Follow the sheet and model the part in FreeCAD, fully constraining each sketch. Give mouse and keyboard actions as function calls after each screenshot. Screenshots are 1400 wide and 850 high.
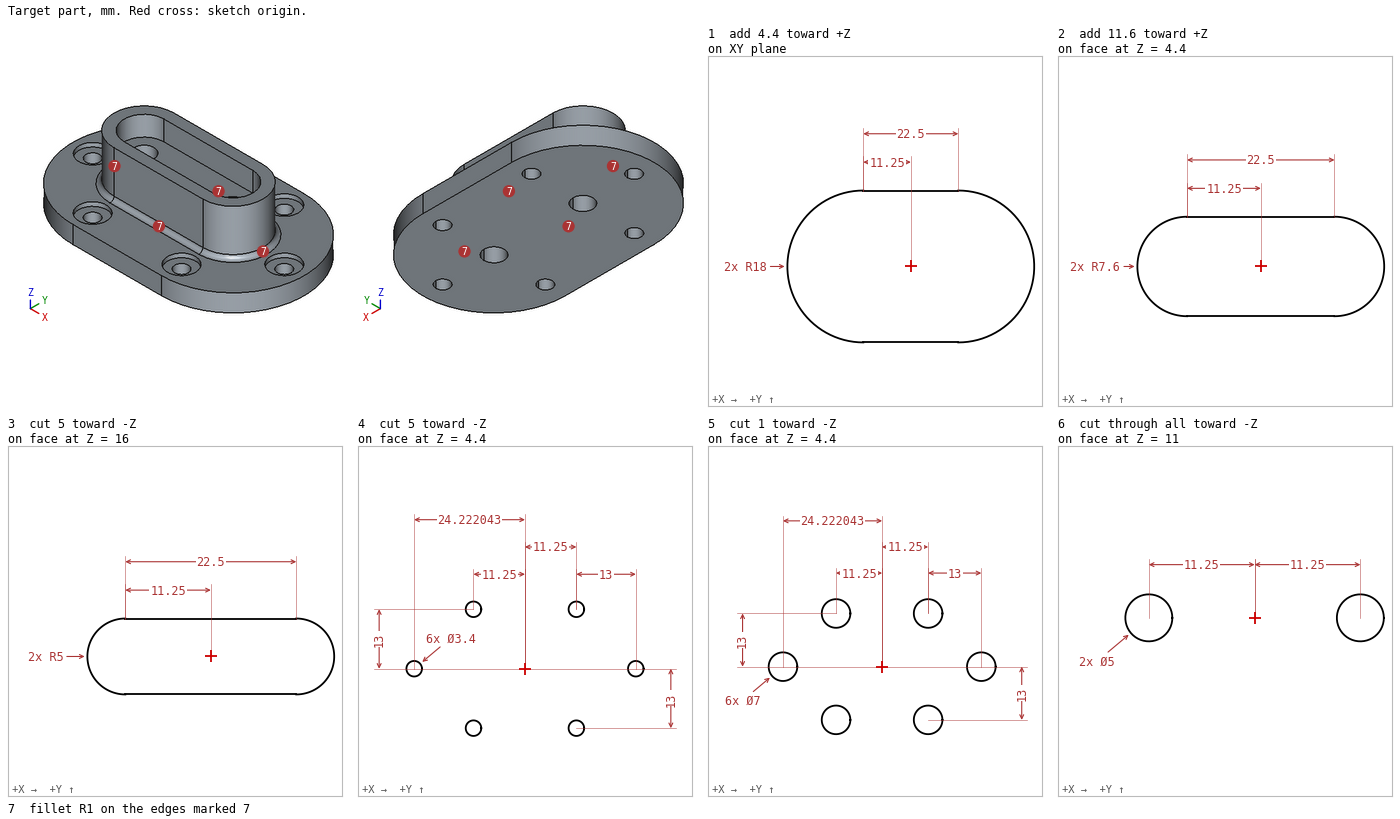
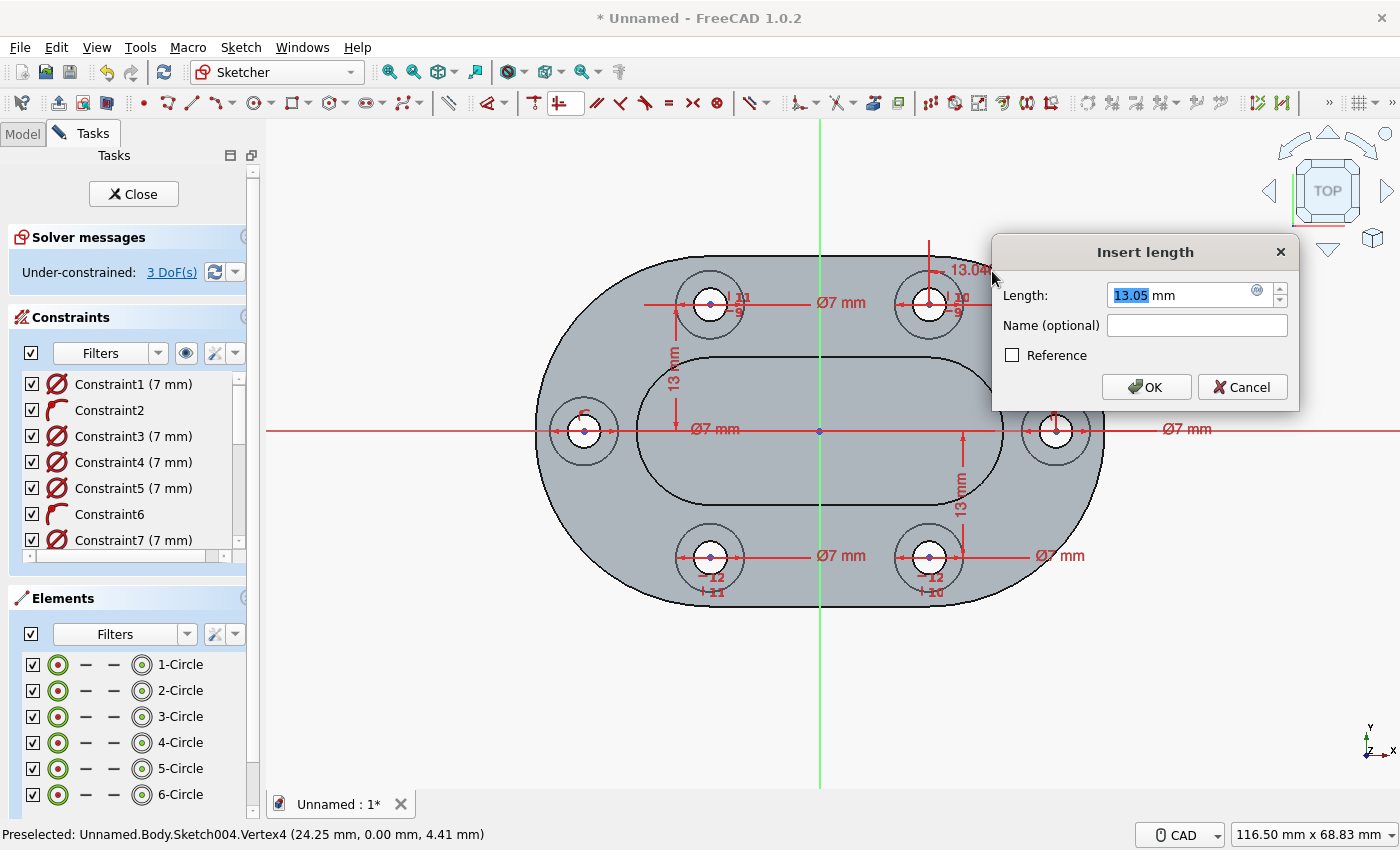
text(13)
key(Return)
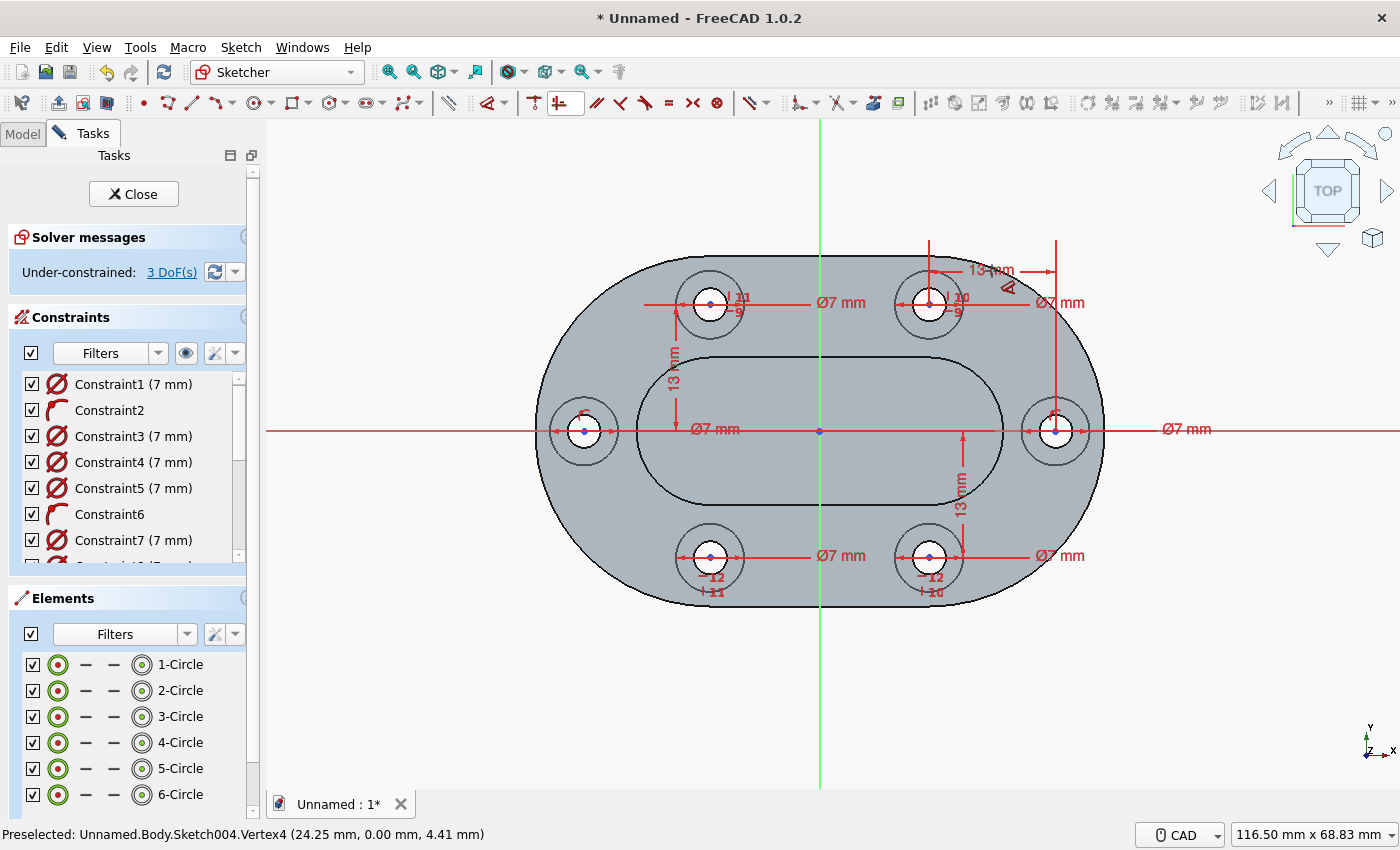
click(710, 305)
click(765, 271)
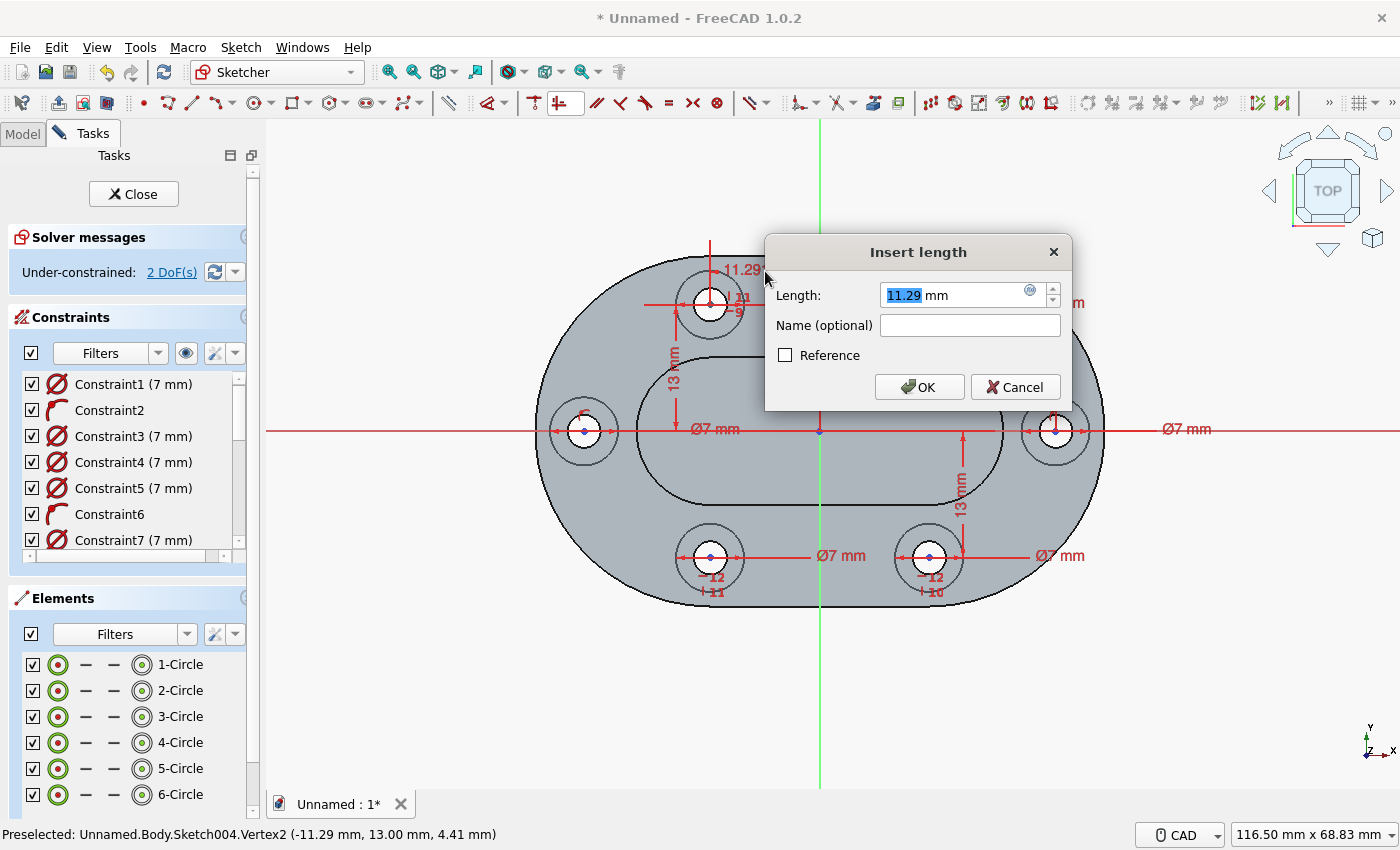
text(11.25)
key(Return)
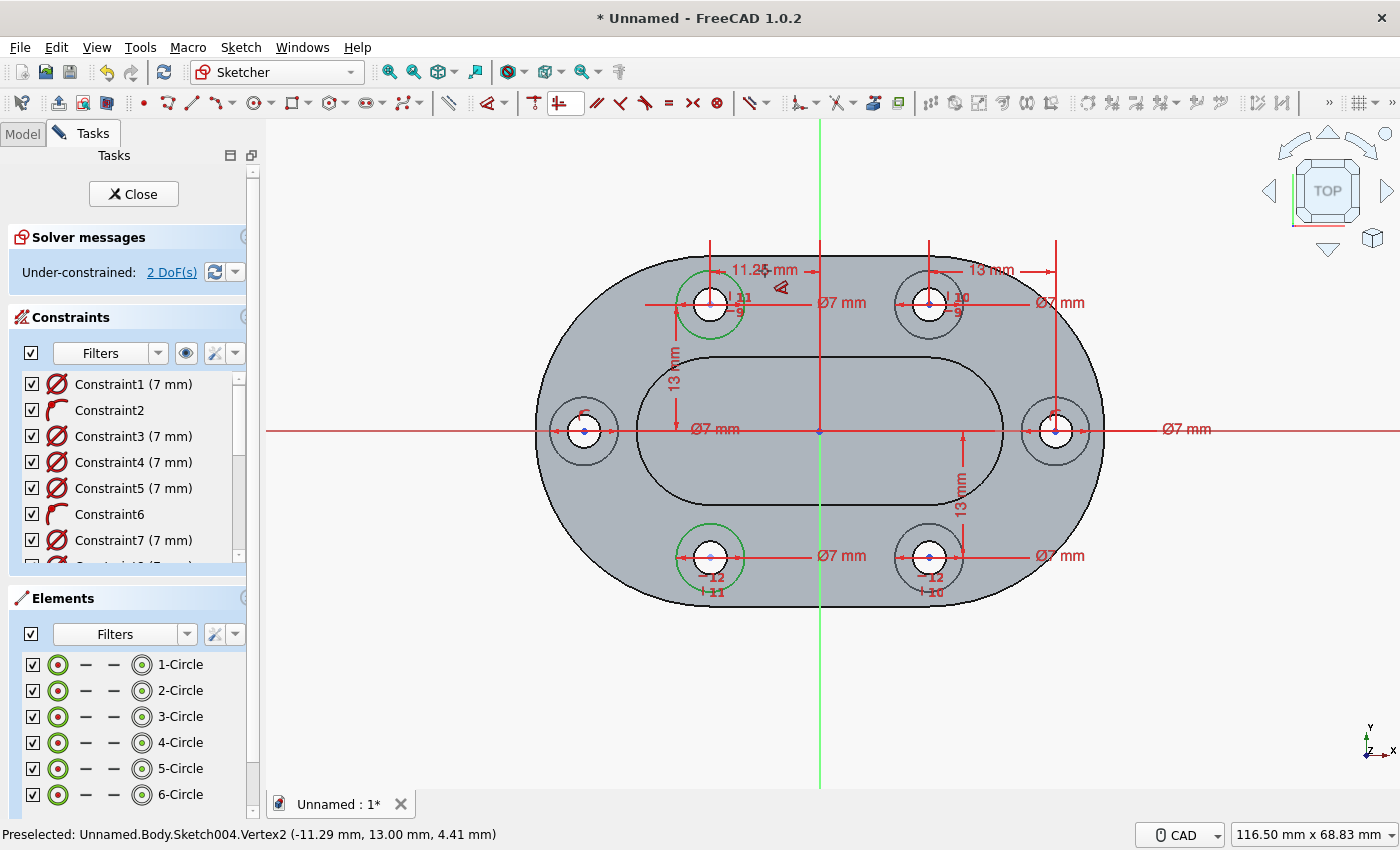
click(929, 305)
click(874, 271)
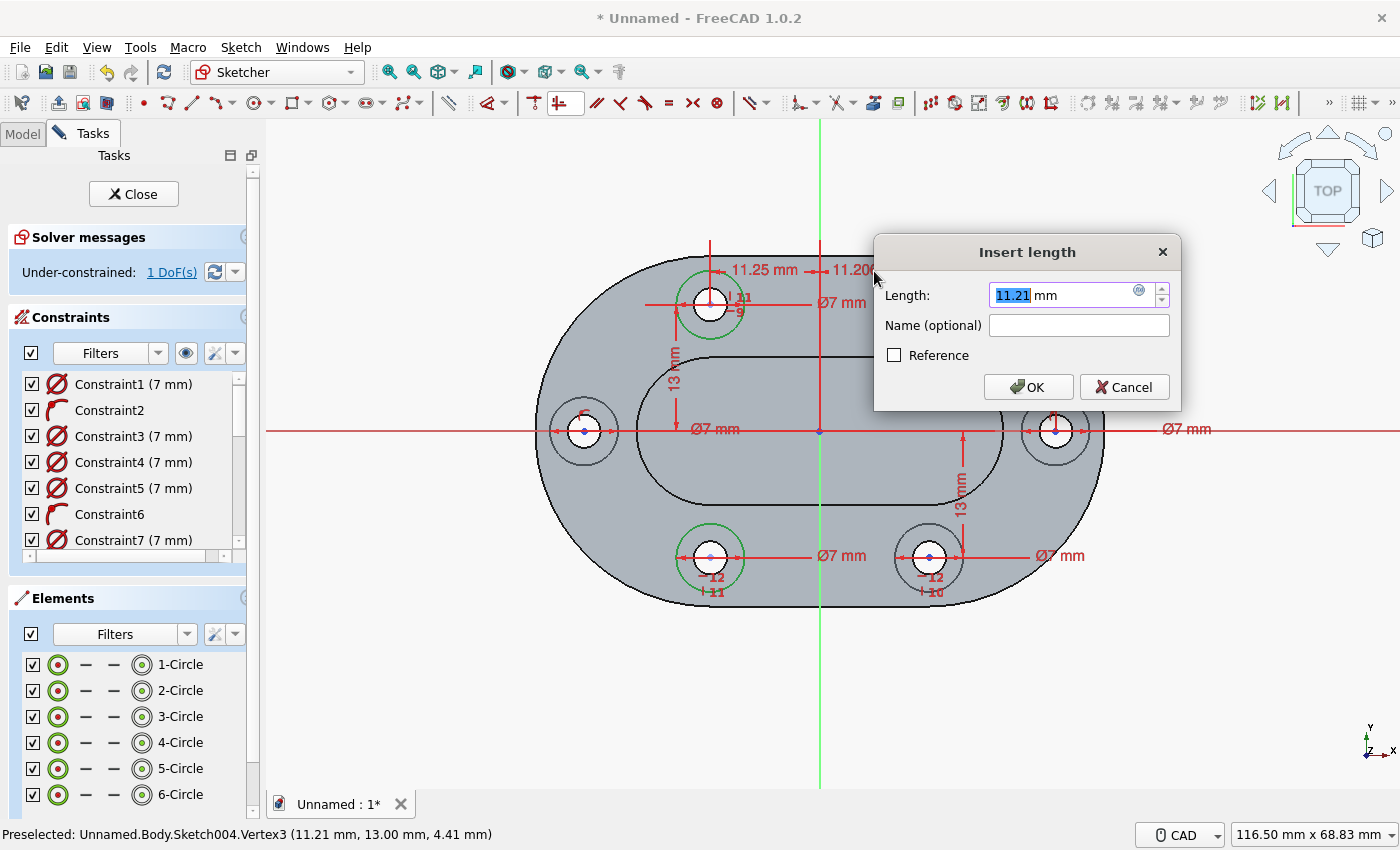
text(11.25)
key(Return)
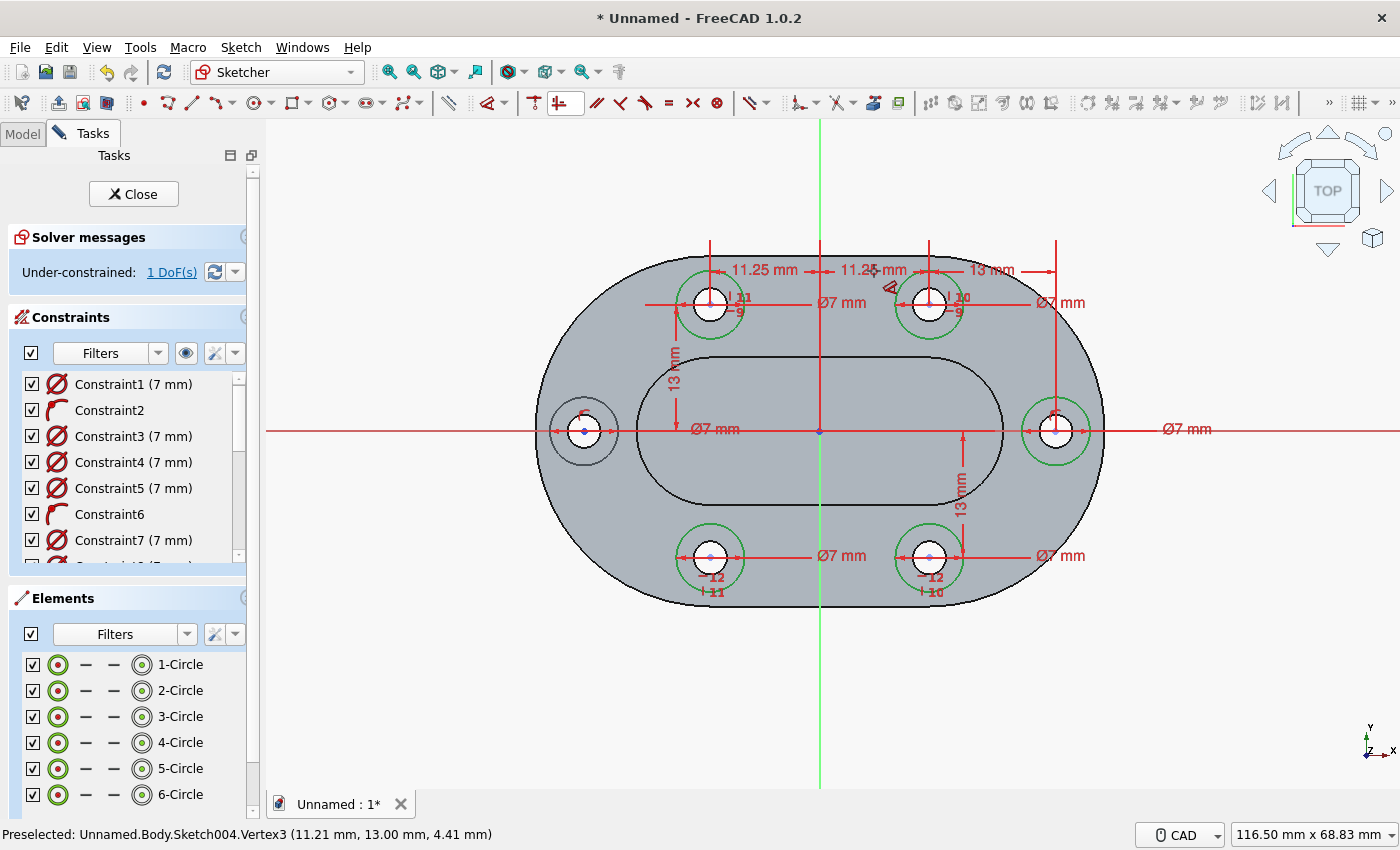
click(584, 431)
click(702, 465)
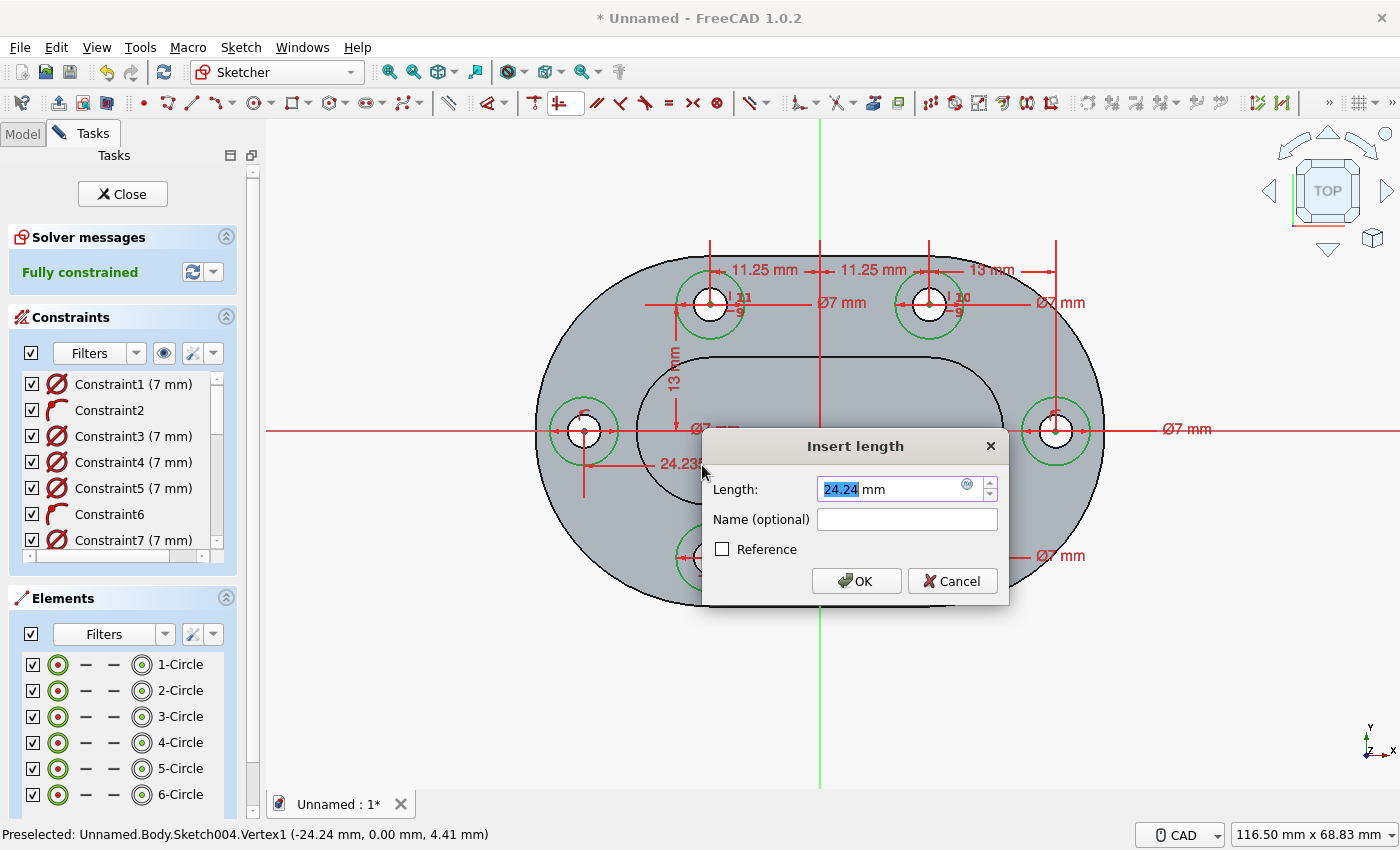
text(24.222043)
key(Return)
key(Escape)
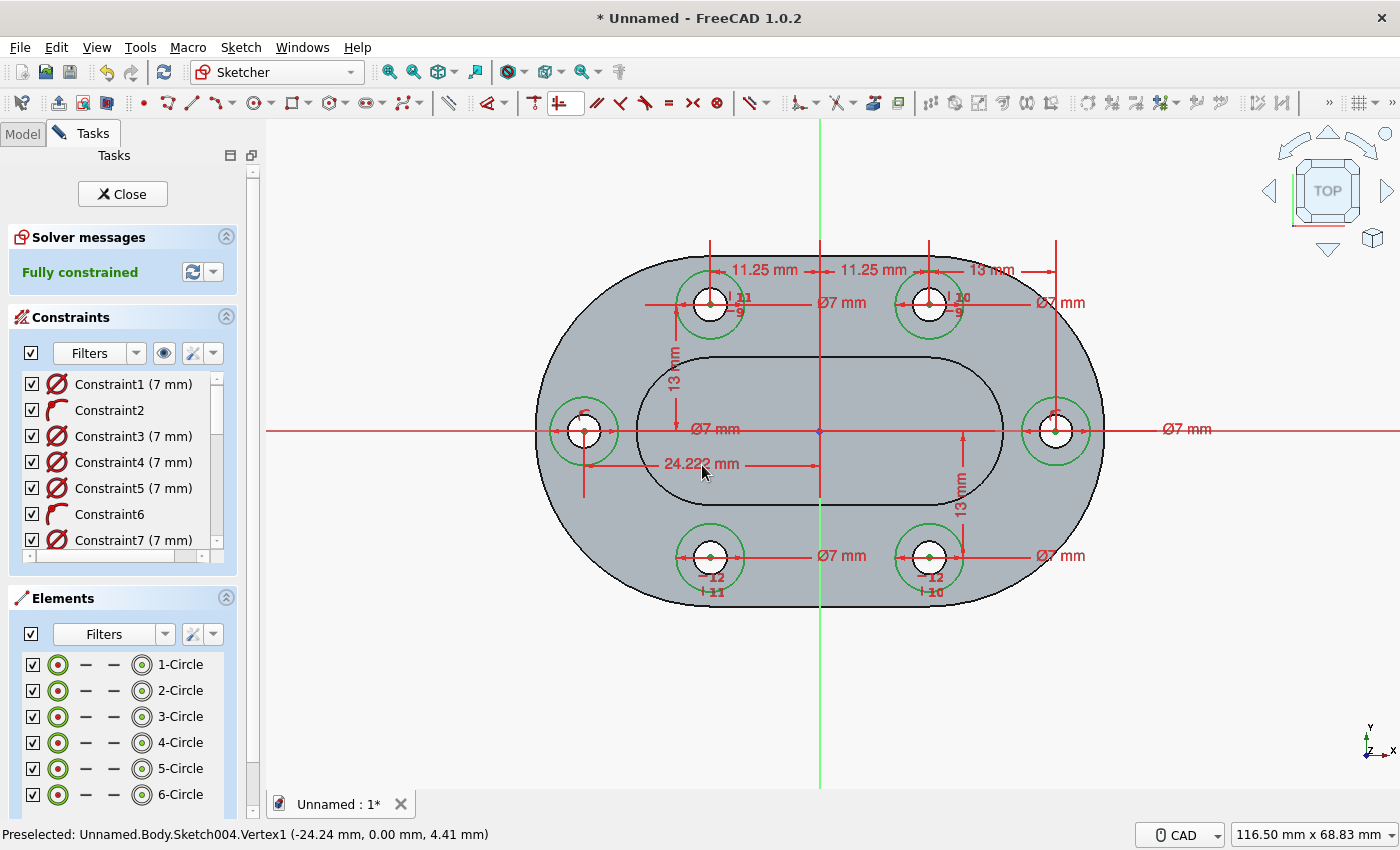
click(123, 194)